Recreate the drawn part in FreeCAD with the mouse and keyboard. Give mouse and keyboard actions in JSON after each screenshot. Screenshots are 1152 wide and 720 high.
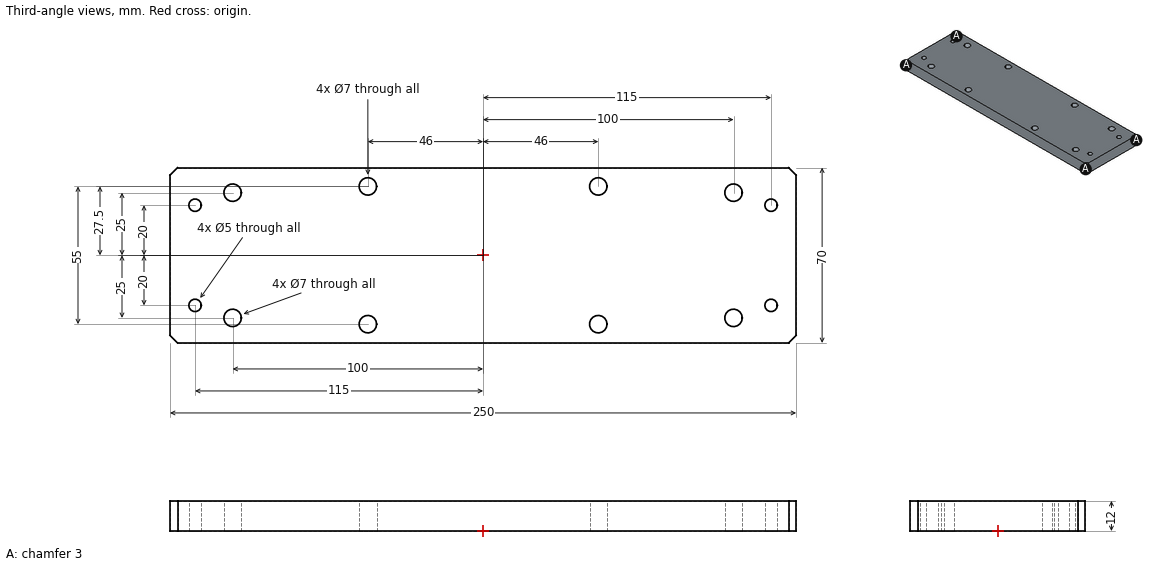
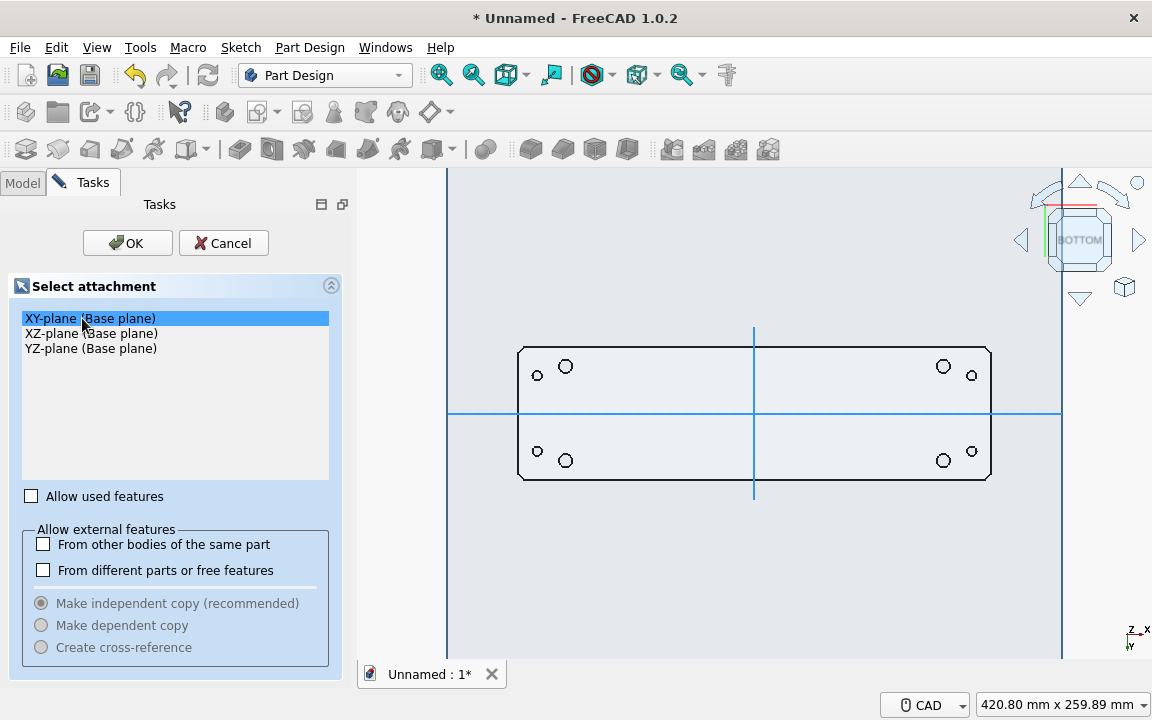
{"action": "left_click", "coordinate": [128, 243]}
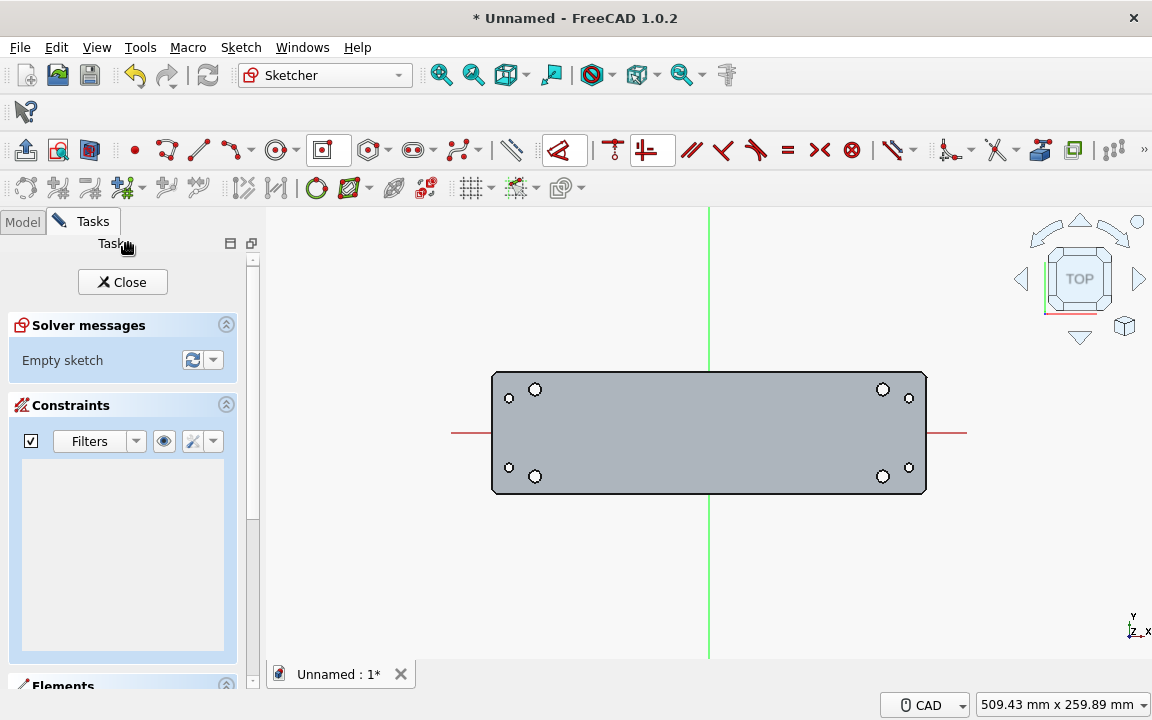
{"action": "key", "text": "q s"}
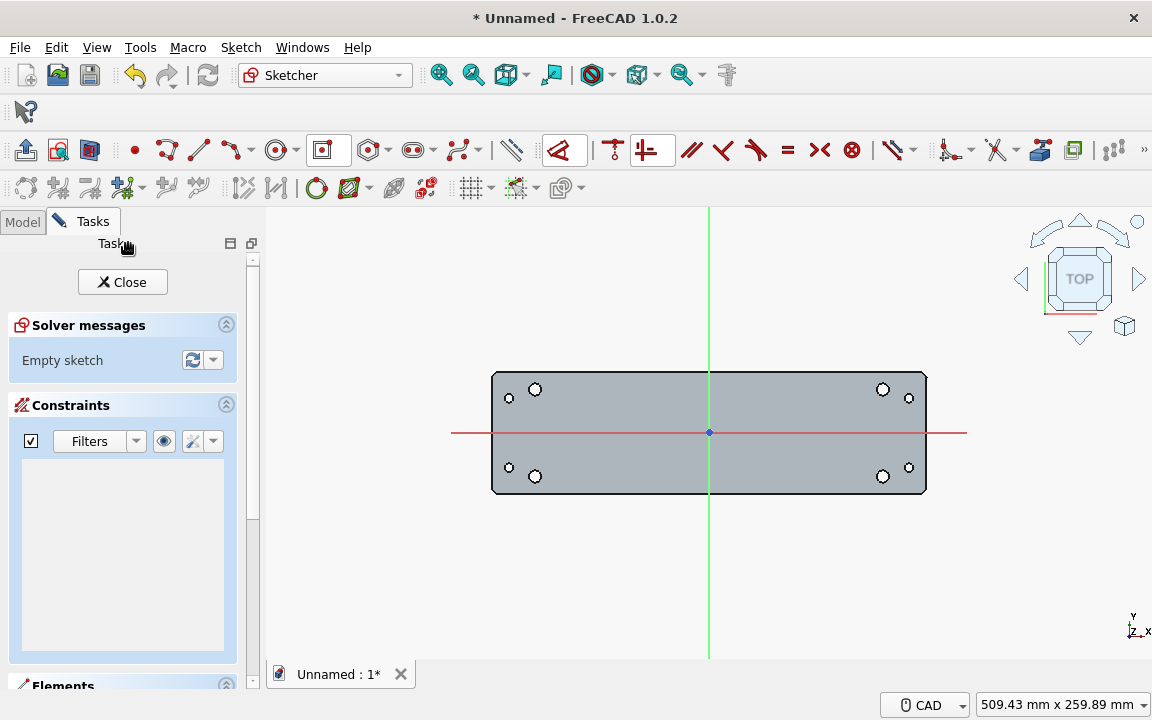
{"action": "scroll", "coordinate": [749, 433], "scroll_direction": "up", "scroll_amount": 5}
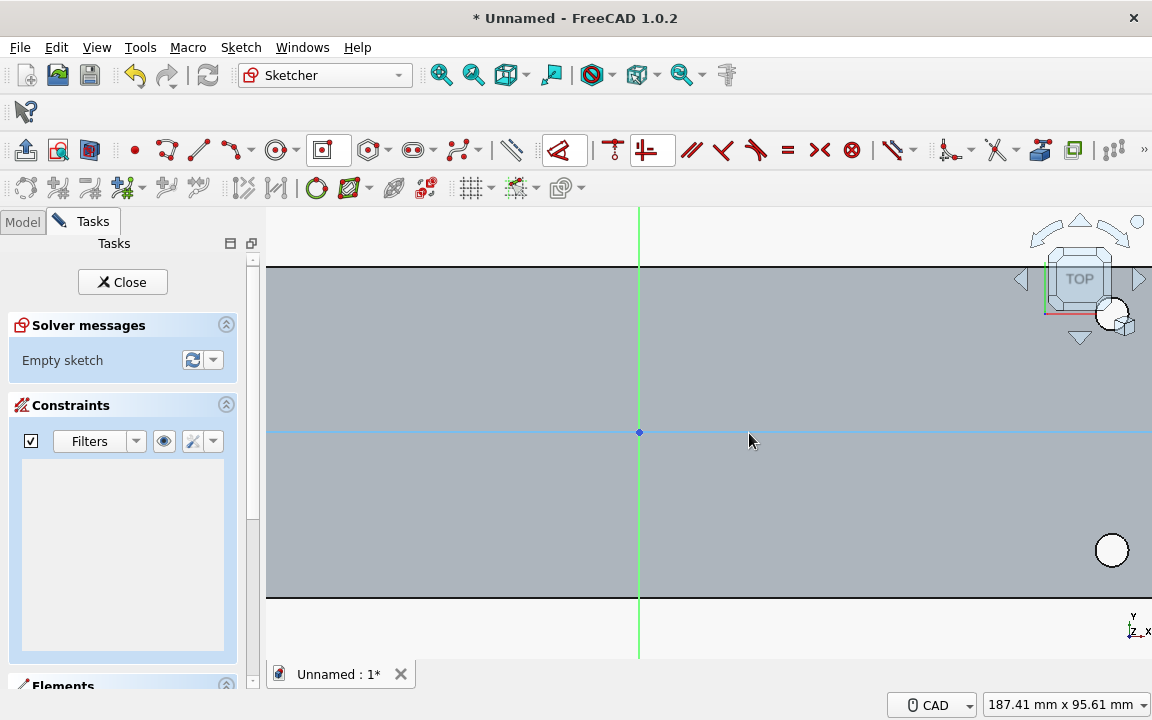
{"action": "left_click", "coordinate": [276, 150]}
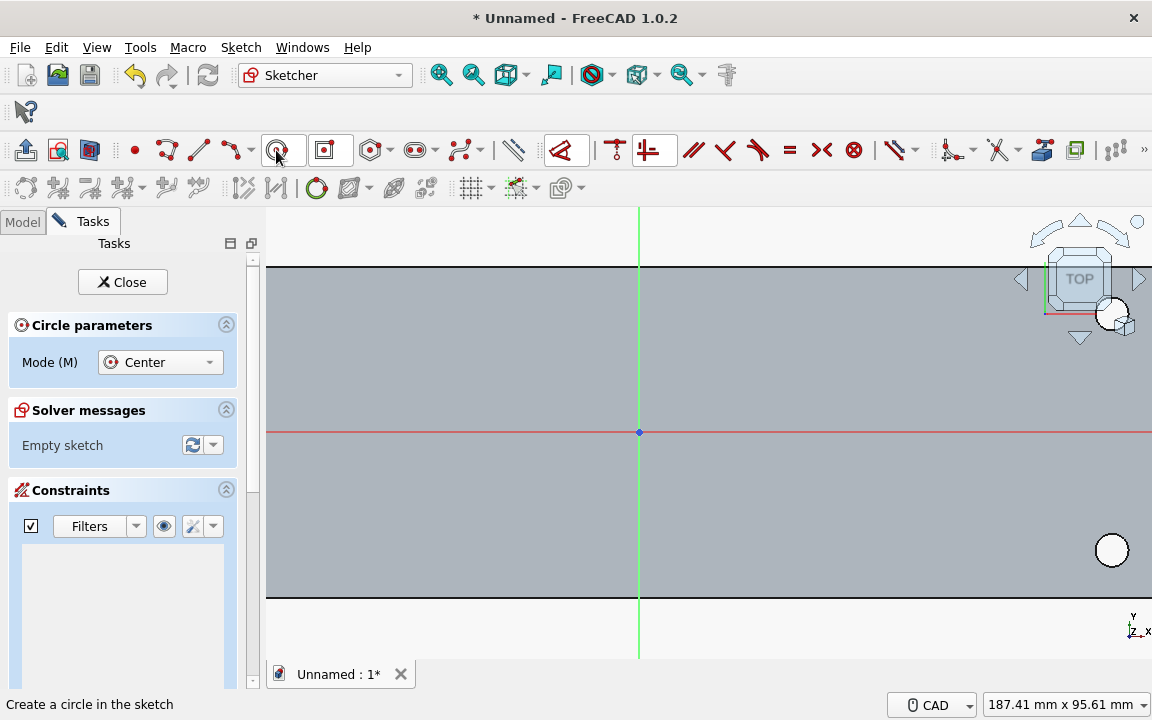
{"action": "scroll", "coordinate": [422, 302], "scroll_direction": "up", "scroll_amount": 2}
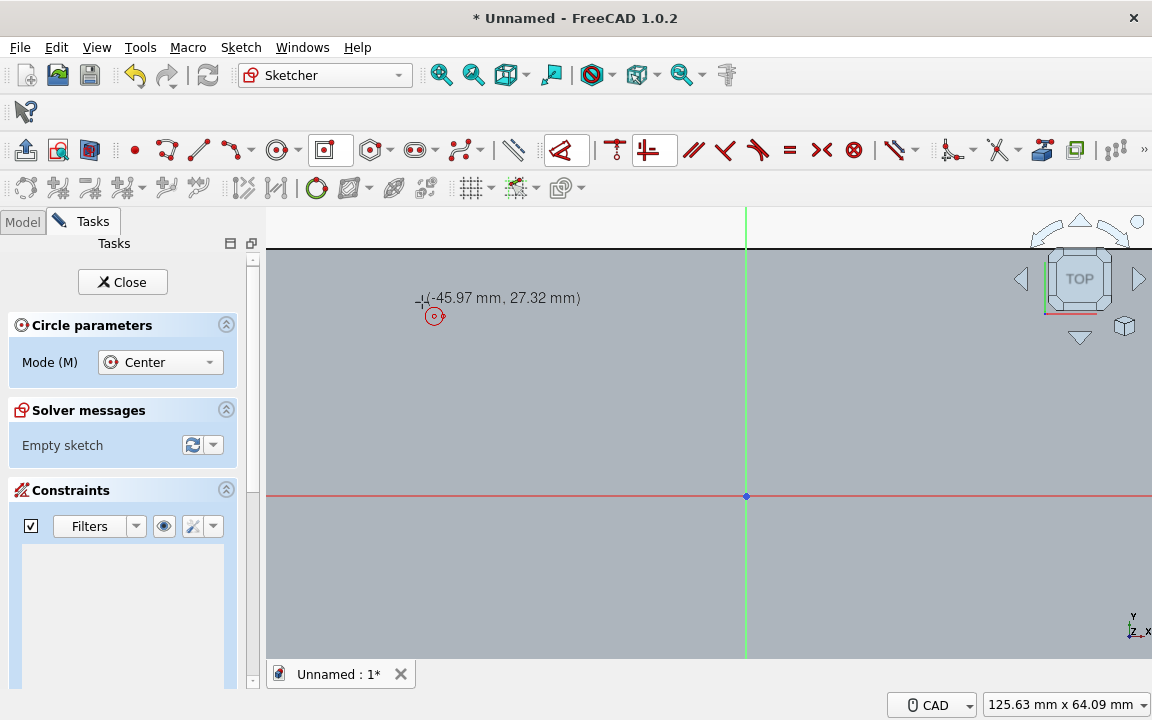
{"action": "left_click", "coordinate": [422, 302]}
{"action": "left_click", "coordinate": [439, 285]}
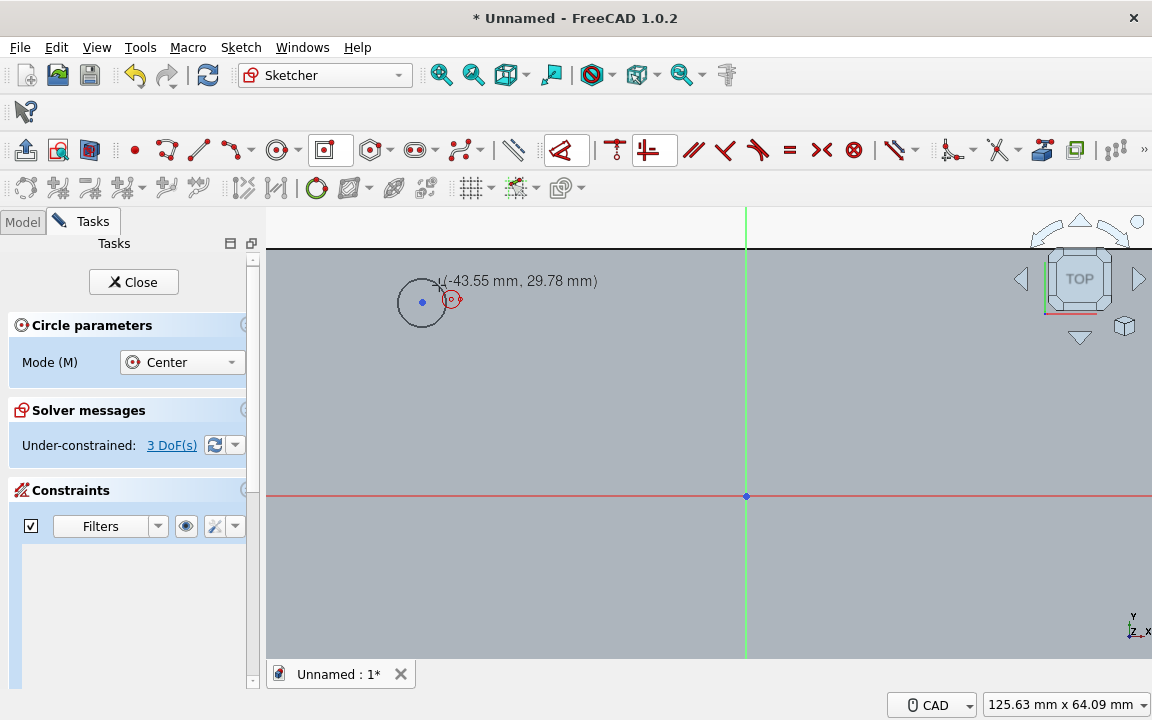
{"action": "scroll", "coordinate": [426, 305], "scroll_direction": "down", "scroll_amount": 2}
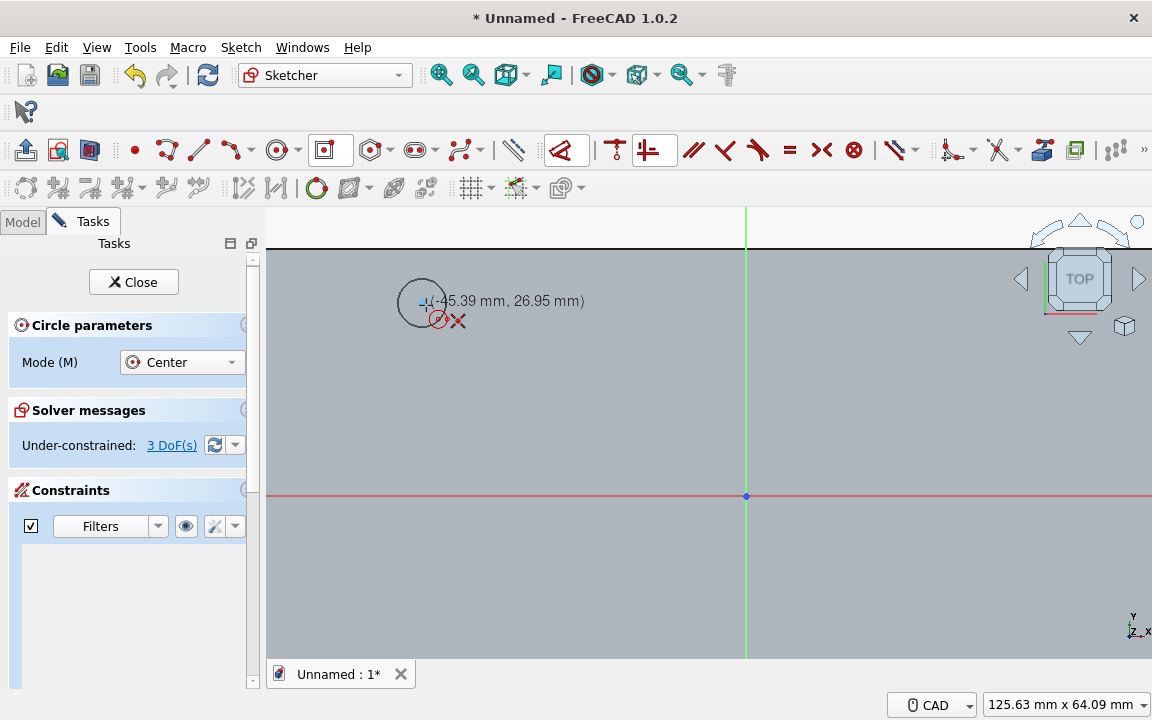
{"action": "scroll", "coordinate": [423, 563], "scroll_direction": "up", "scroll_amount": 2}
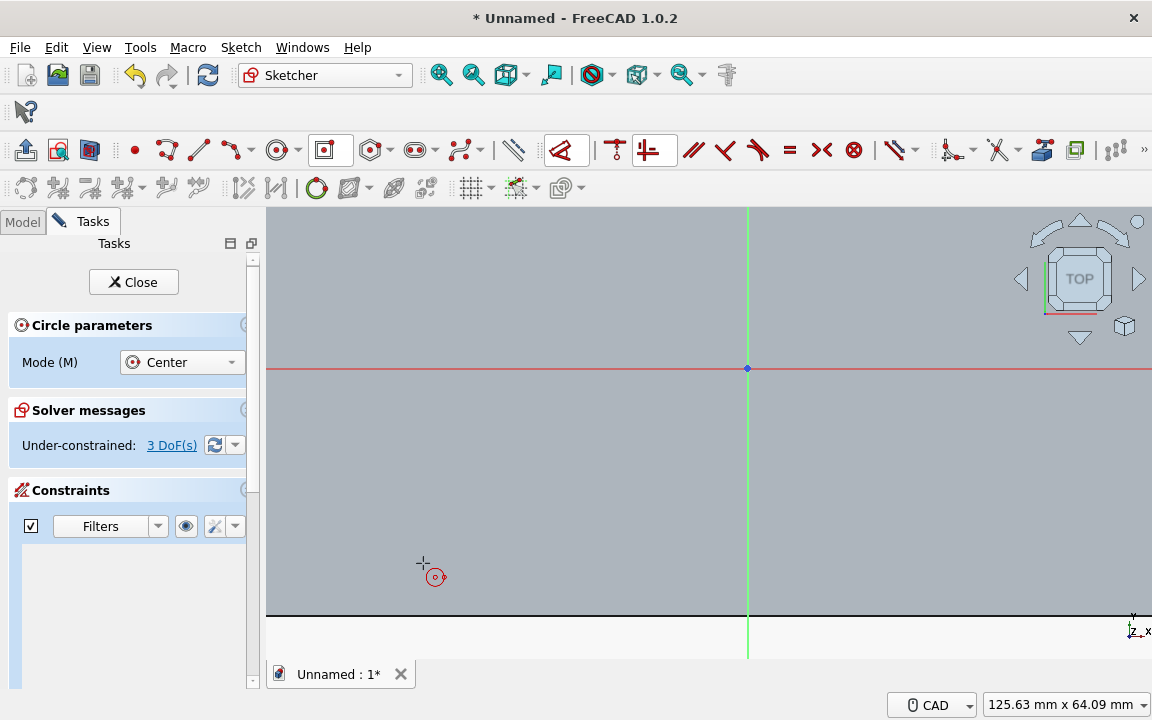
{"action": "left_click", "coordinate": [423, 563]}
{"action": "left_click", "coordinate": [441, 545]}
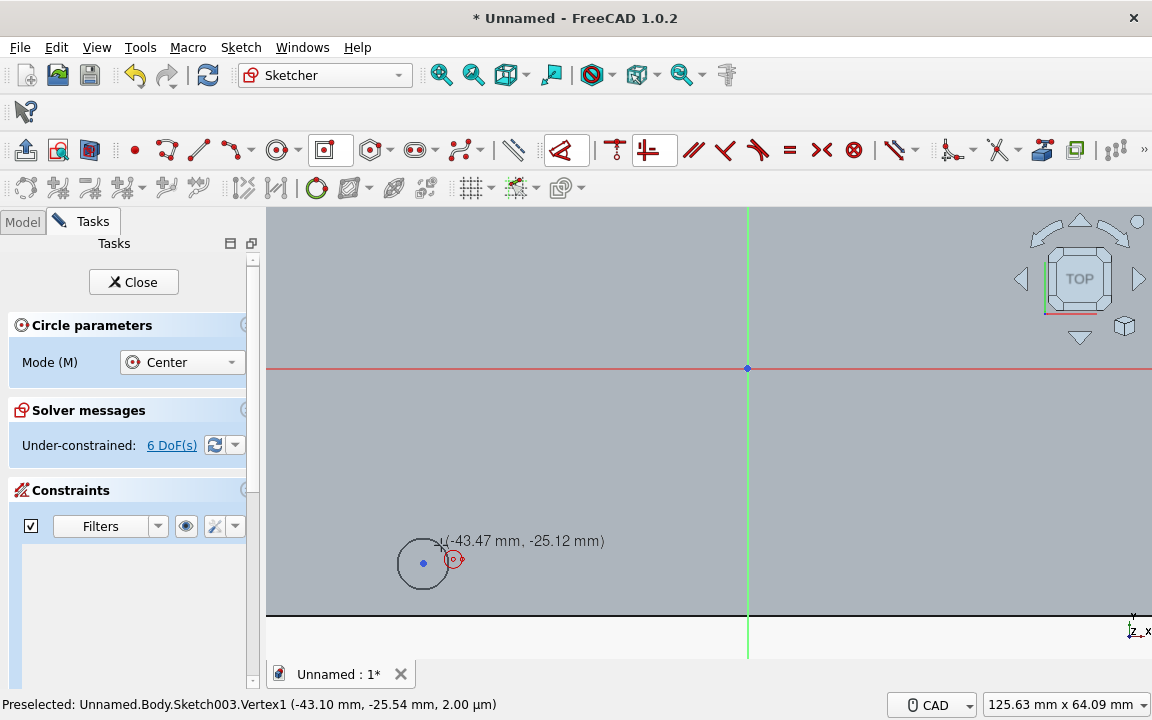
{"action": "scroll", "coordinate": [423, 563], "scroll_direction": "down", "scroll_amount": 2}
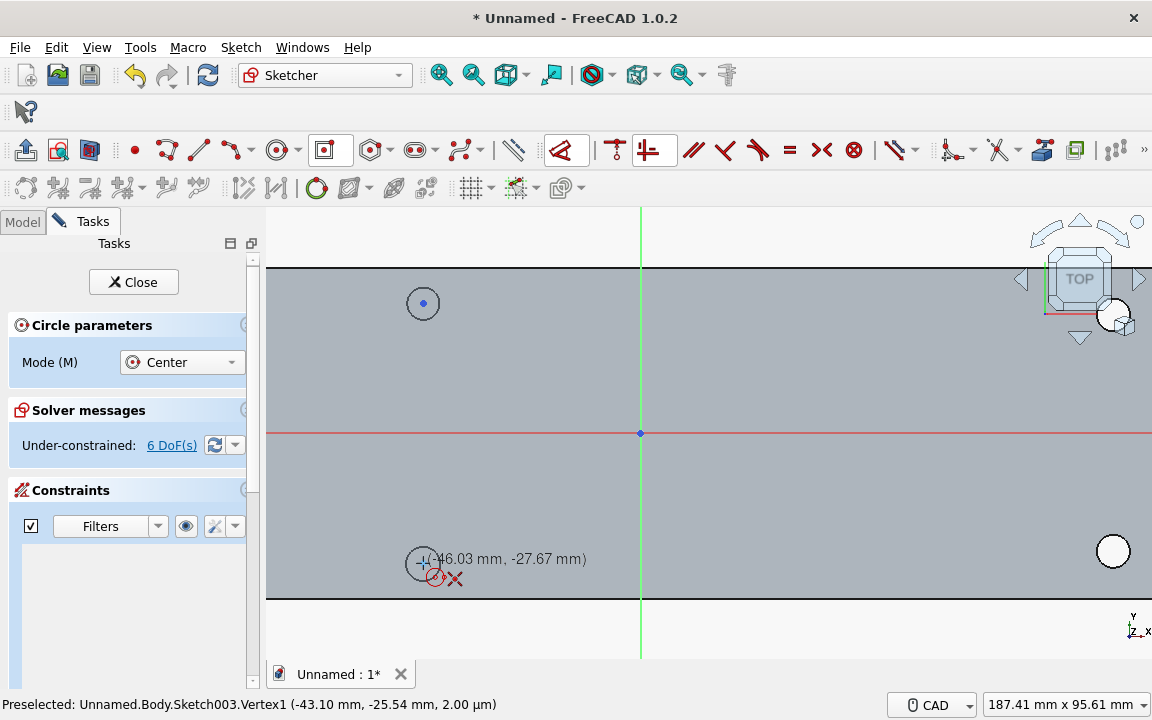
{"action": "scroll", "coordinate": [858, 303], "scroll_direction": "up", "scroll_amount": 2}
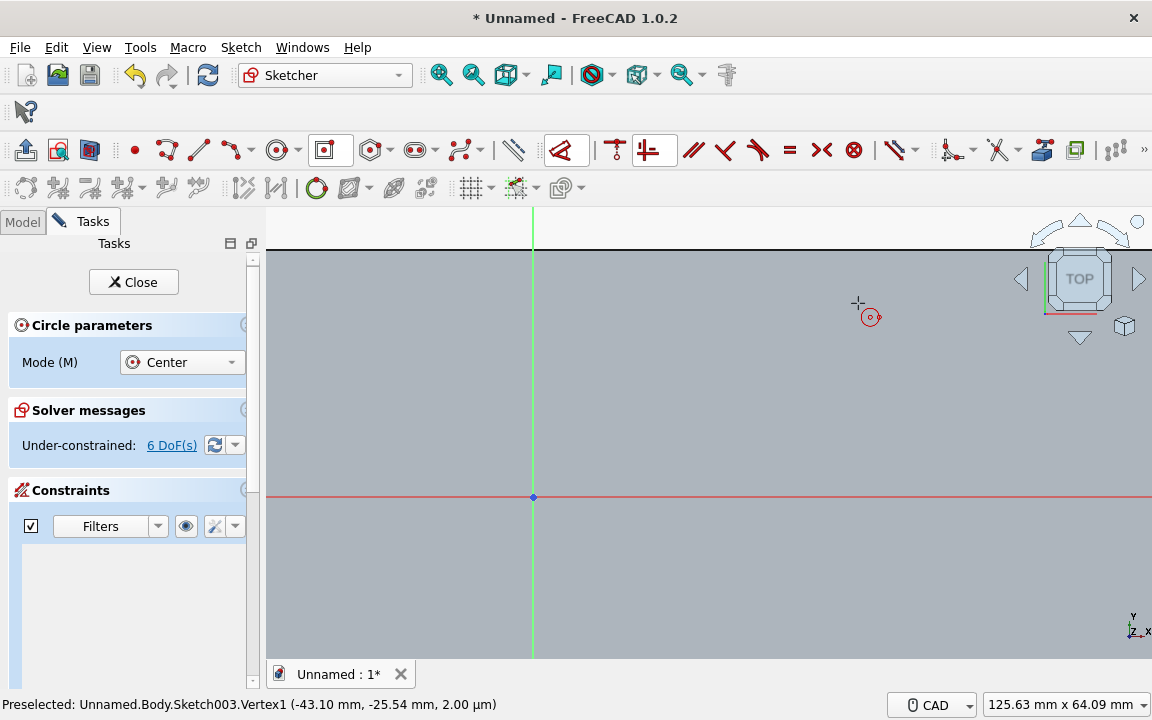
{"action": "left_click", "coordinate": [858, 303]}
{"action": "left_click", "coordinate": [875, 286]}